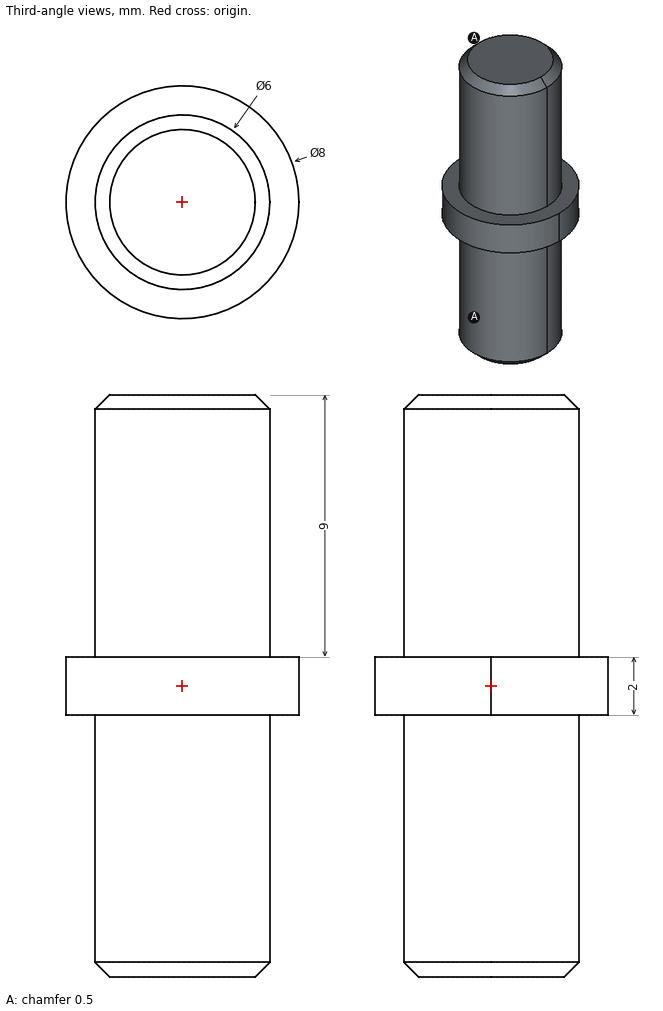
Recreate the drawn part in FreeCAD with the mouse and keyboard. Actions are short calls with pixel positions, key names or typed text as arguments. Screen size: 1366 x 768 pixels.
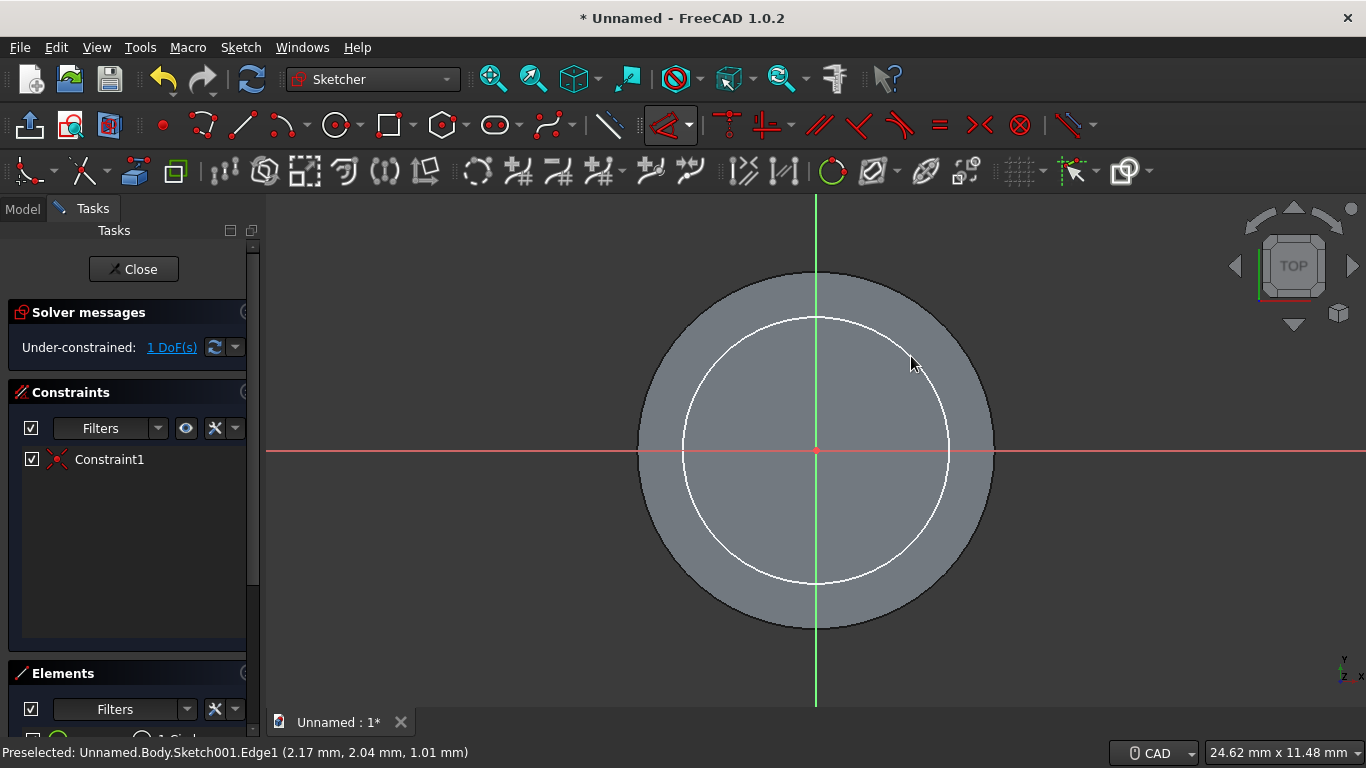
click(664, 126)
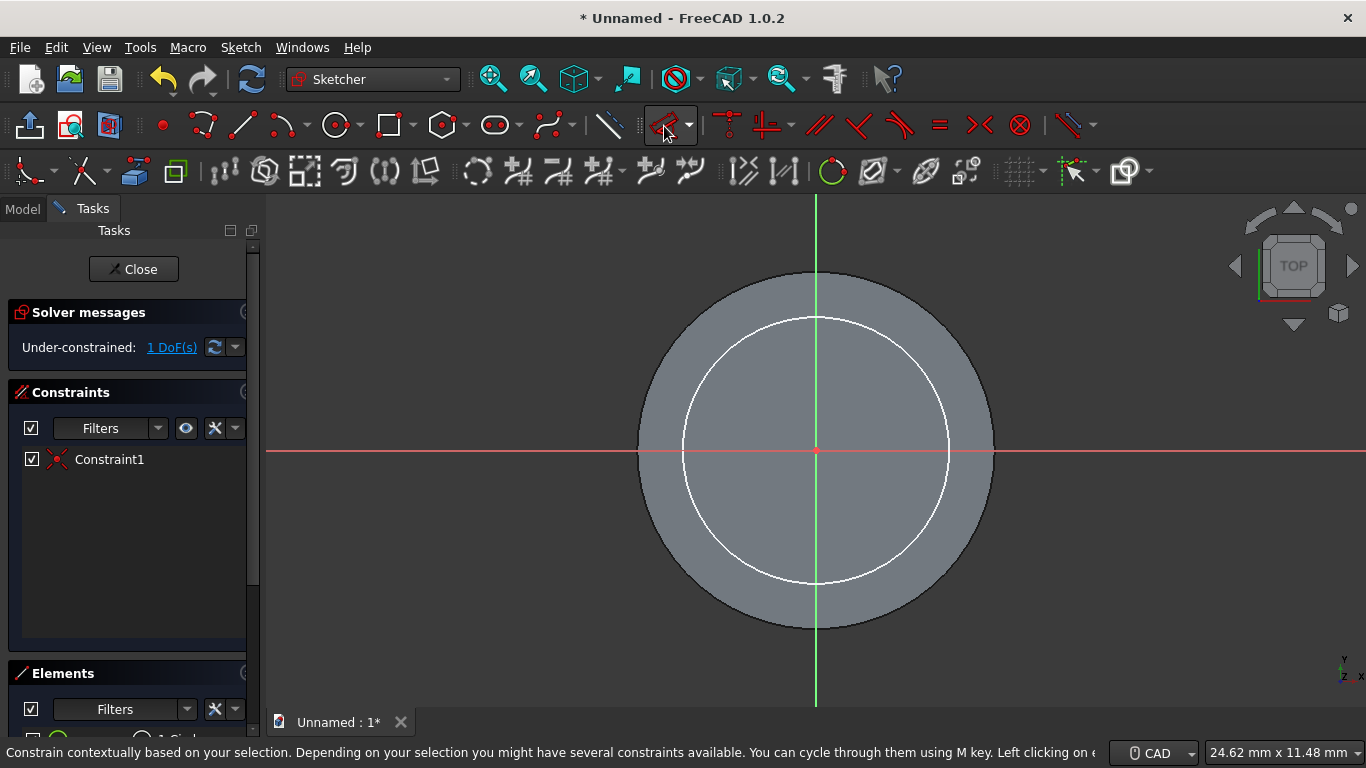
click(910, 356)
click(933, 333)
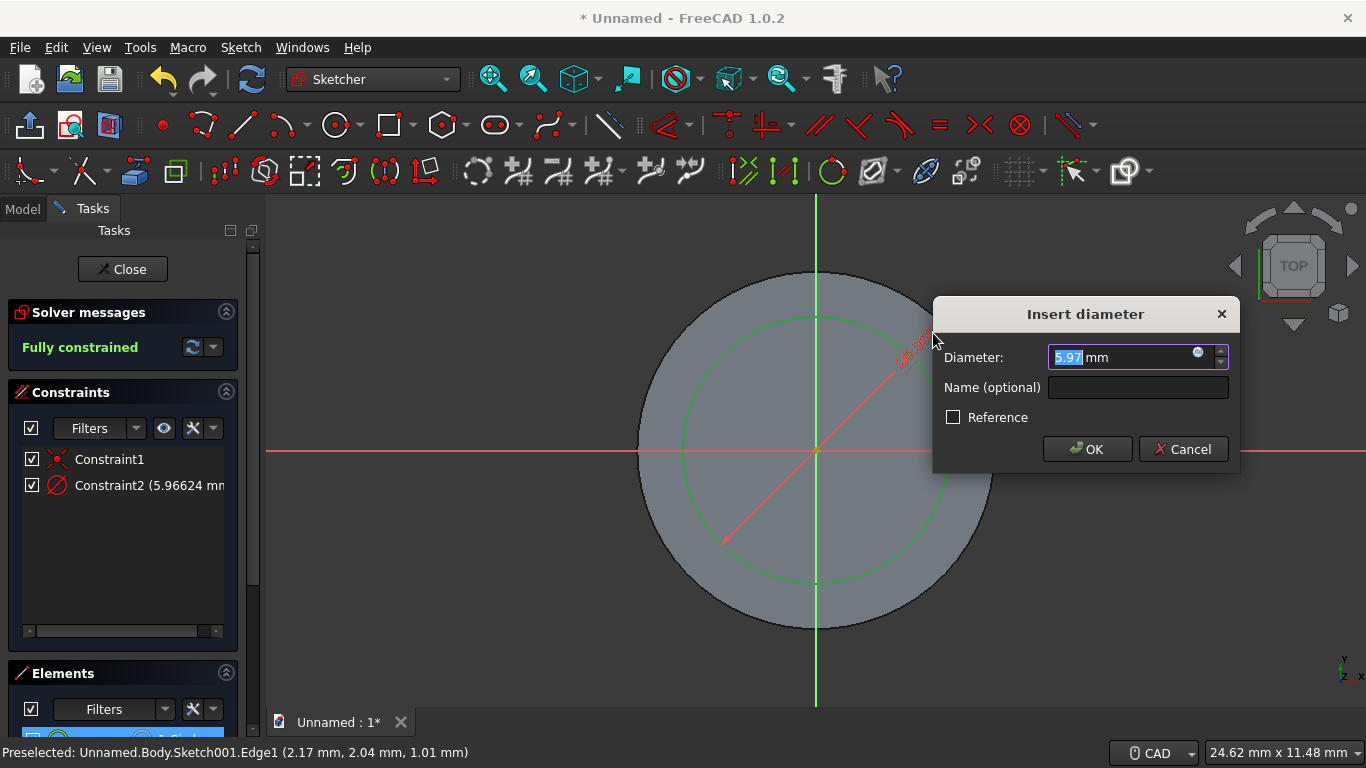
text(6)
key(Return)
key(Escape)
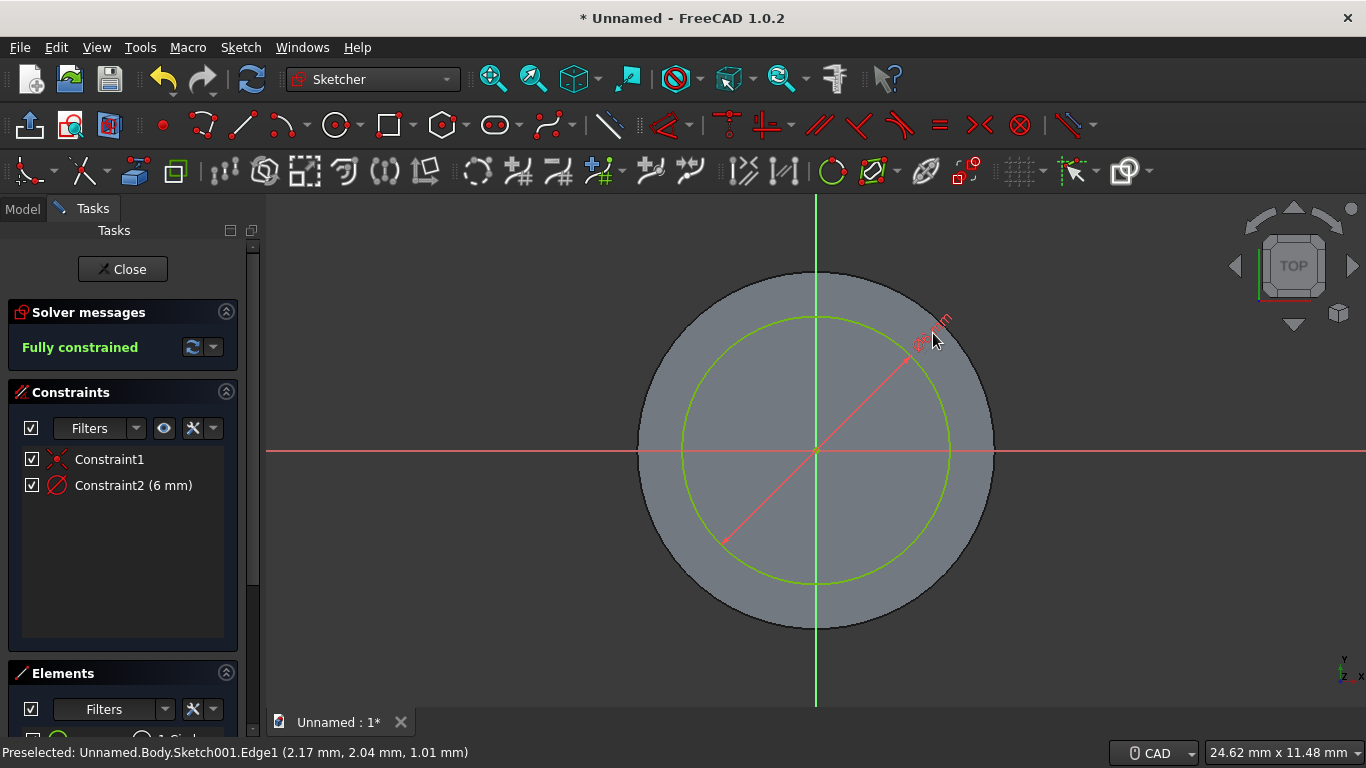
click(123, 269)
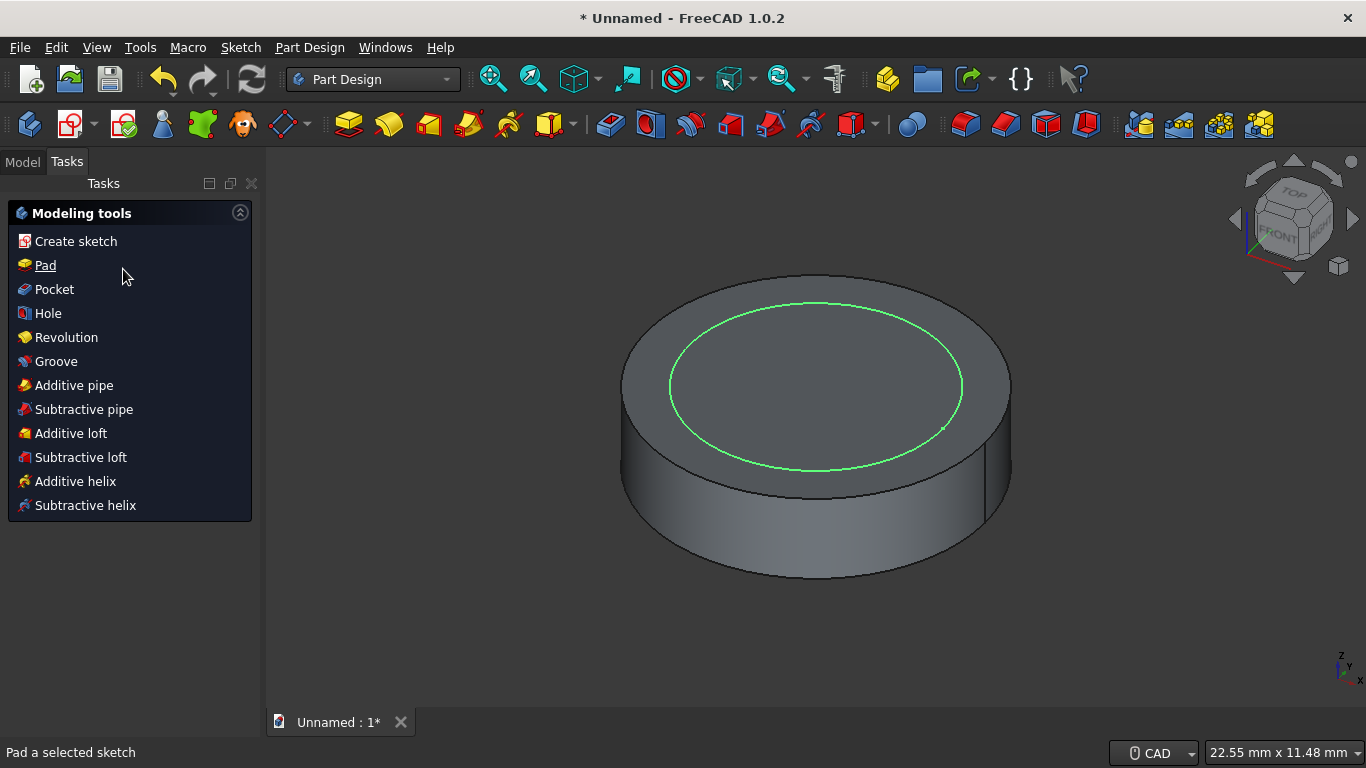
click(350, 124)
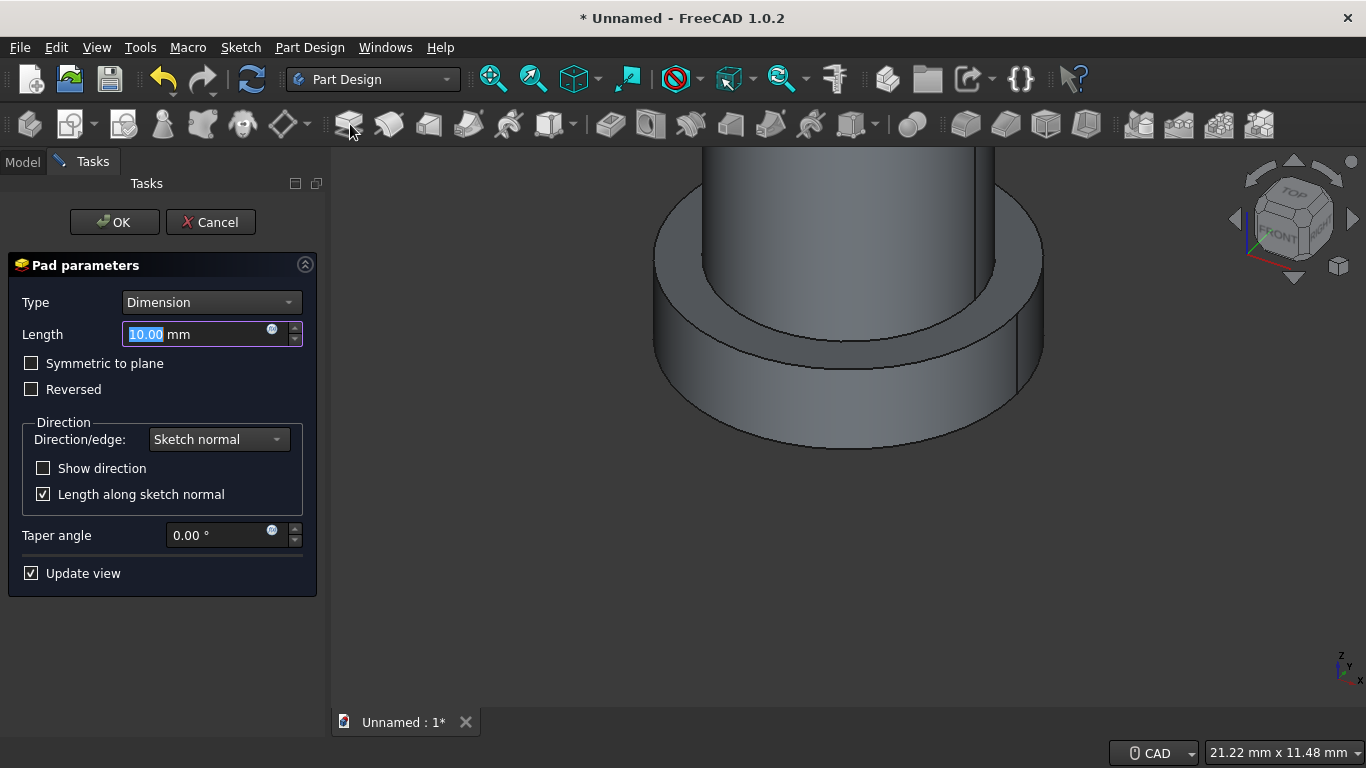
text(9)
key(Tab)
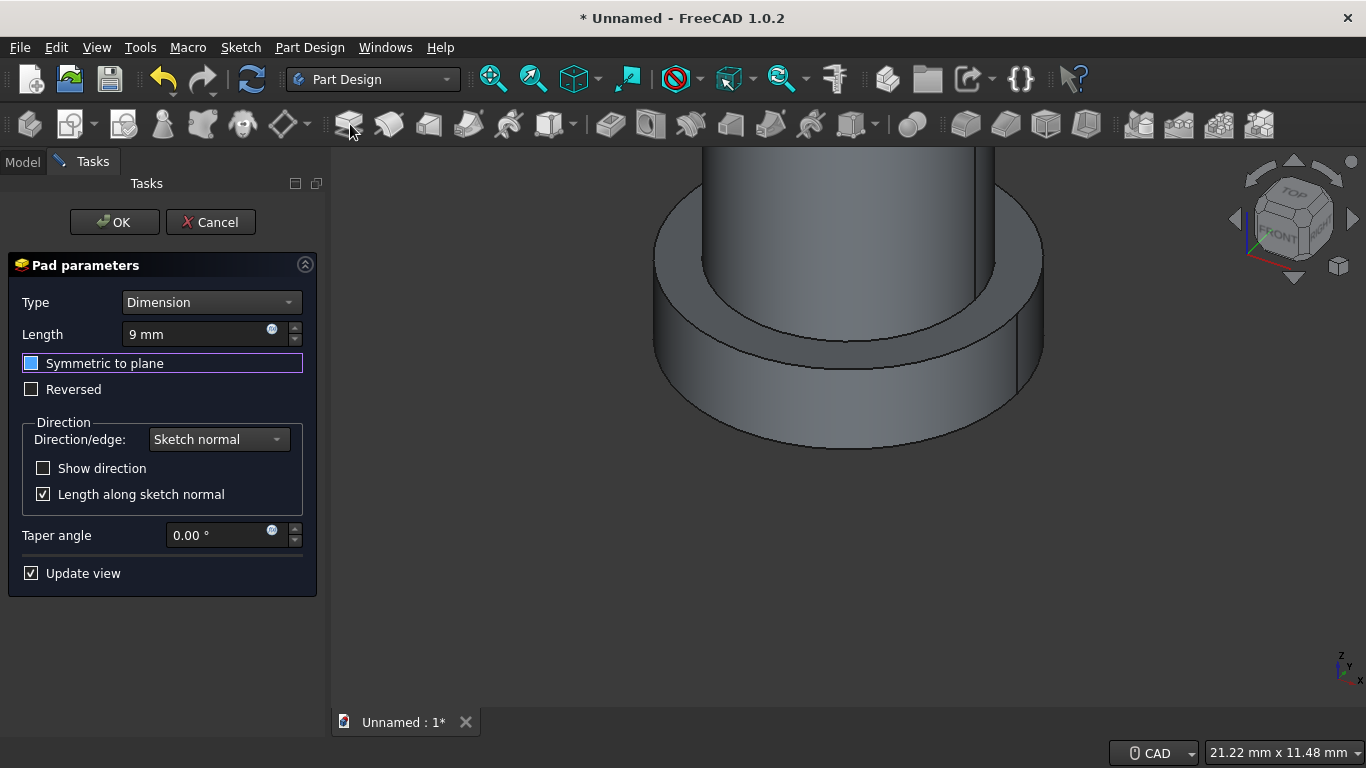
click(115, 222)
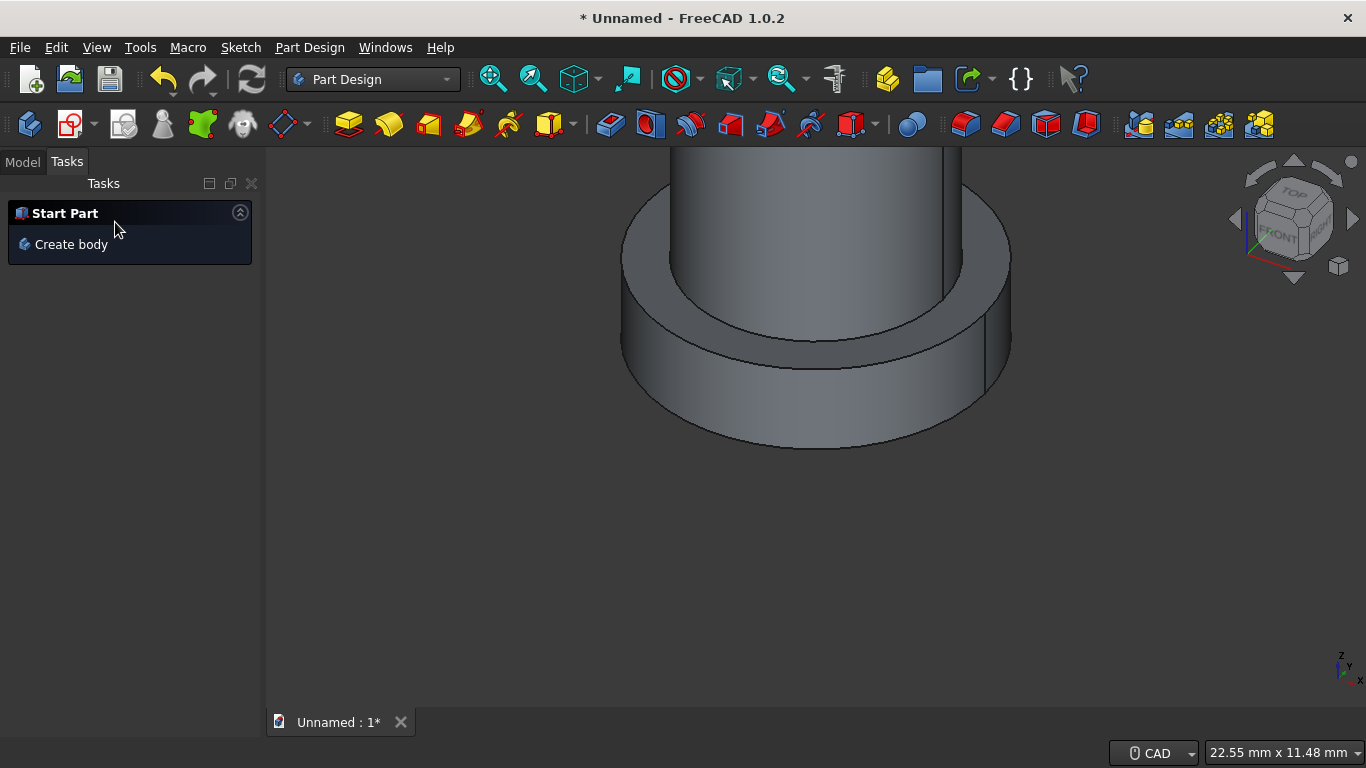
key(v)
key(f)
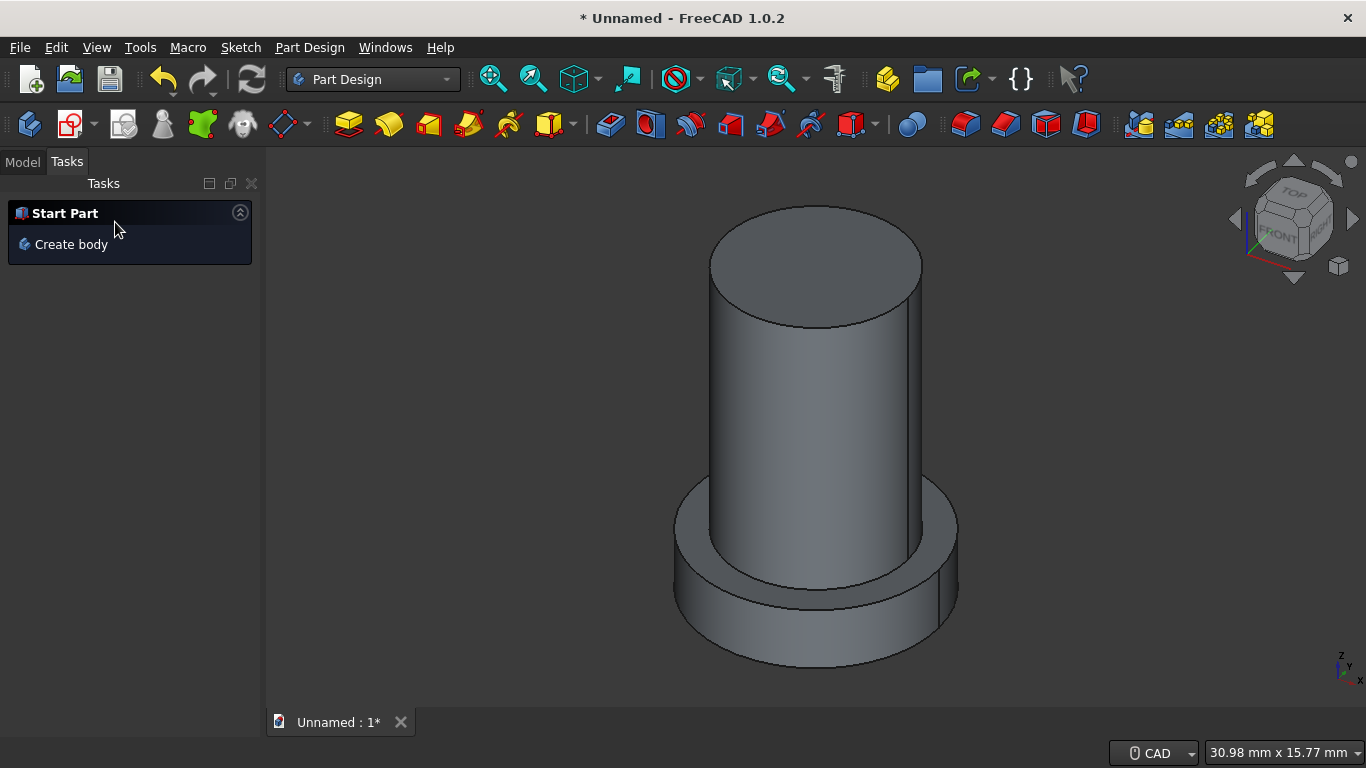
click(23, 161)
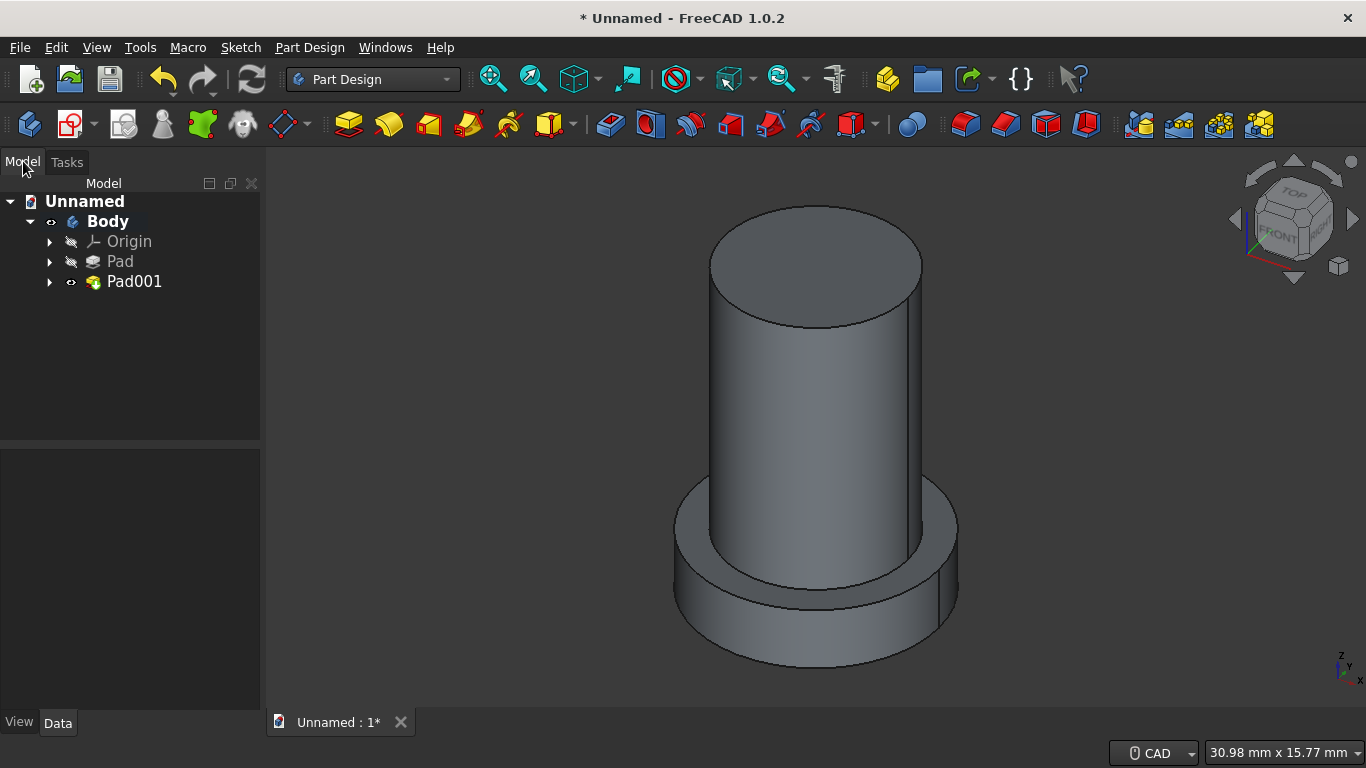
click(116, 282)